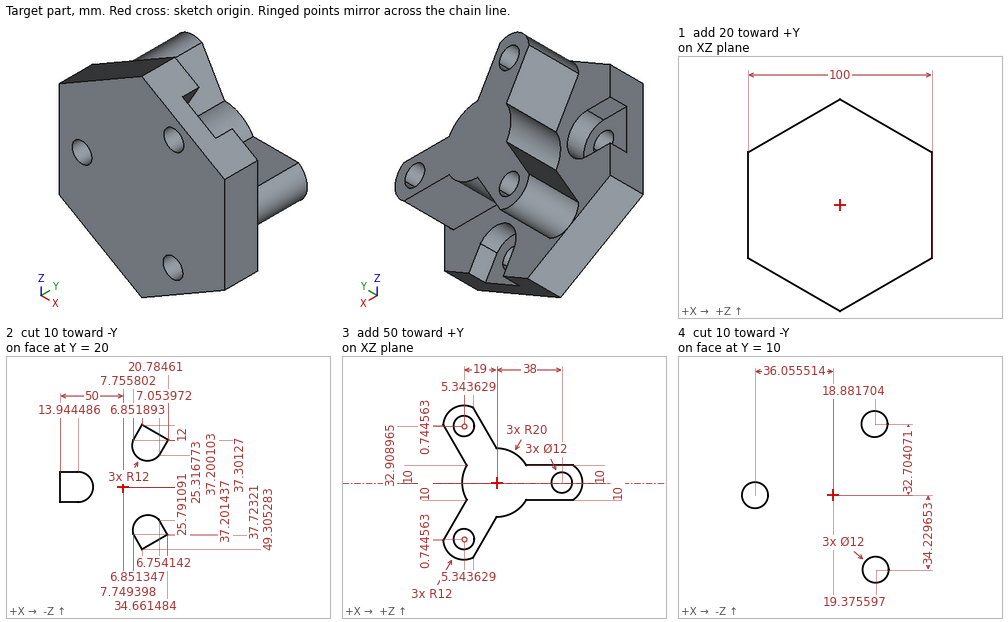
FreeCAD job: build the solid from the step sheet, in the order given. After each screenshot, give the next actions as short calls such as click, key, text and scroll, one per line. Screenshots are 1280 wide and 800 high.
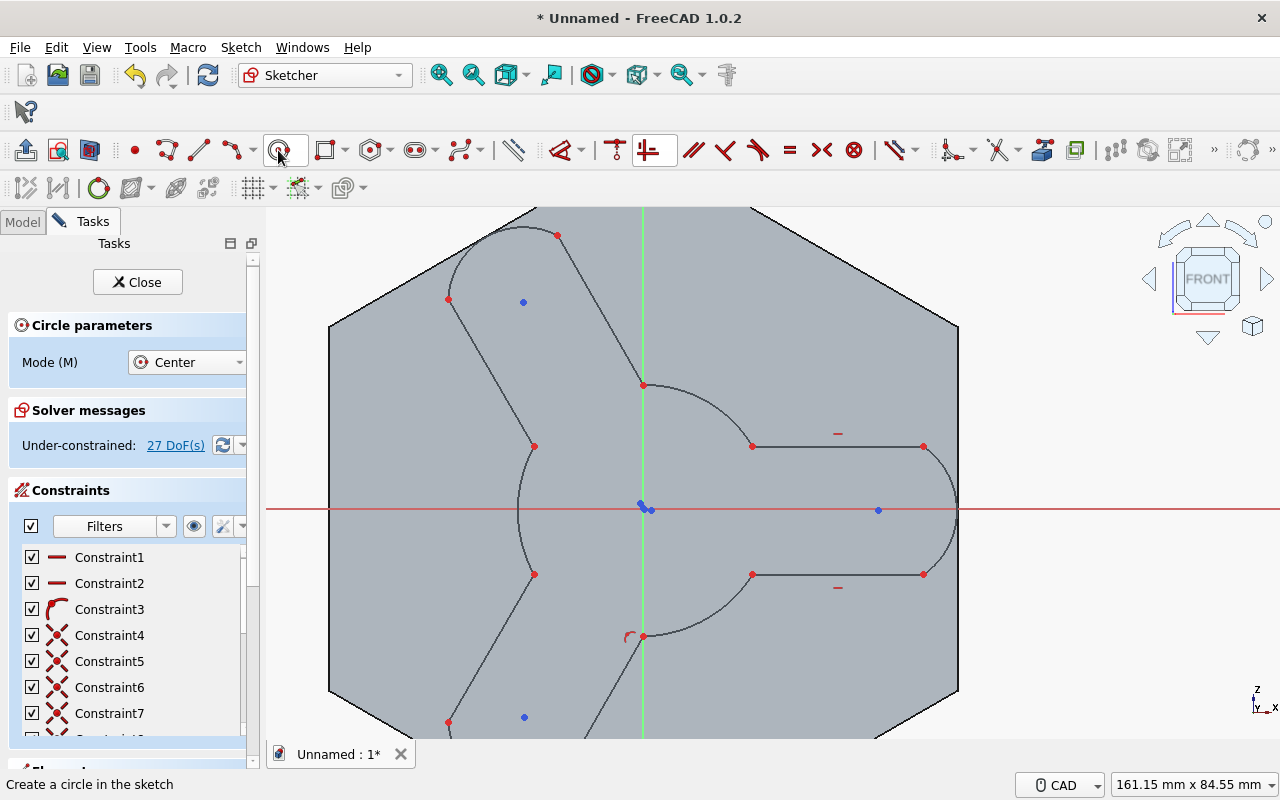
click(524, 302)
move(550, 275)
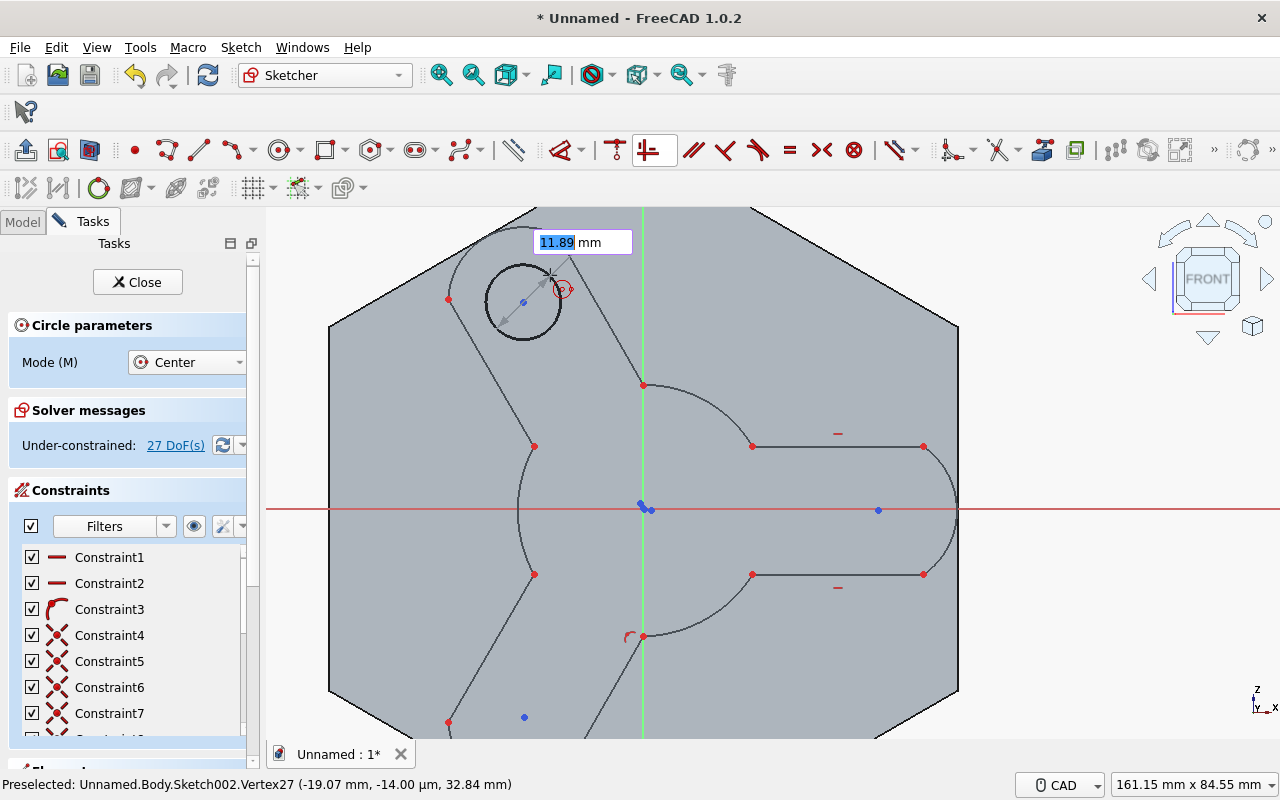
text(12)
key(Return)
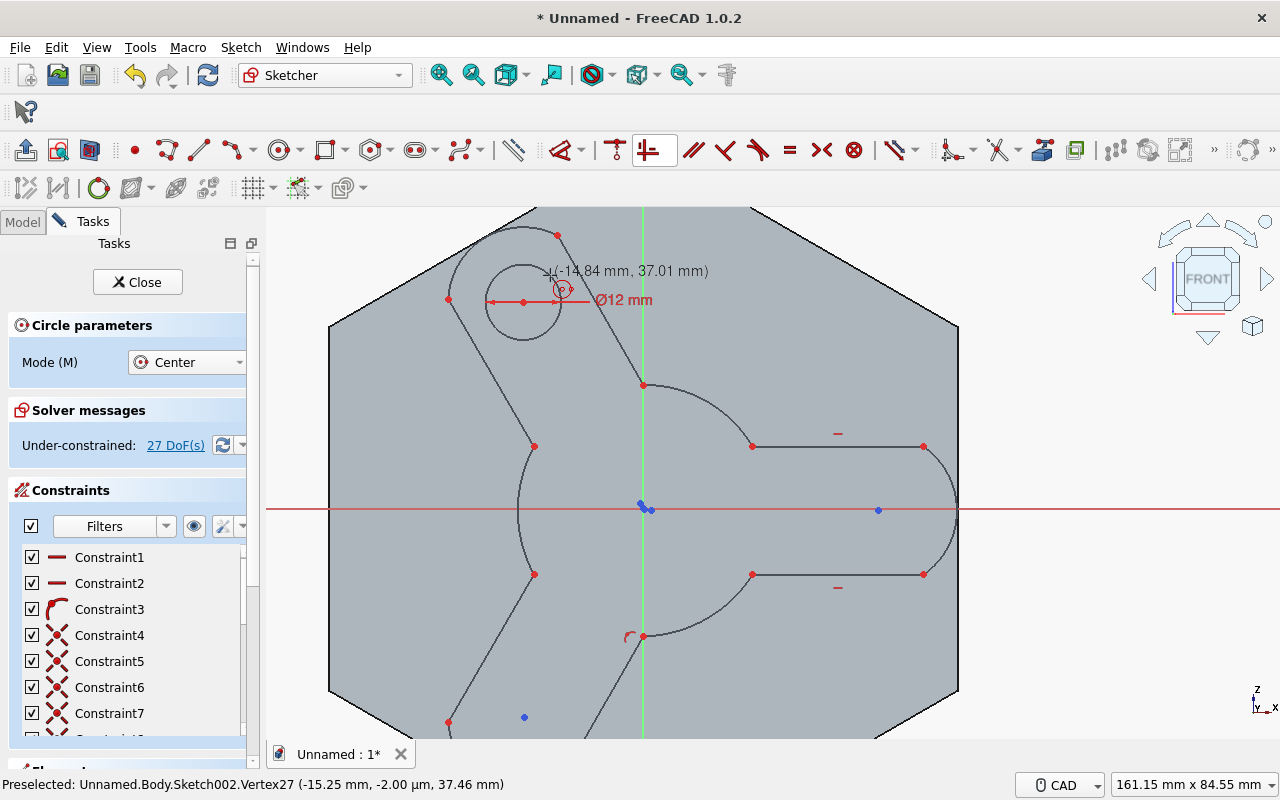
scroll(707, 400, down, 2)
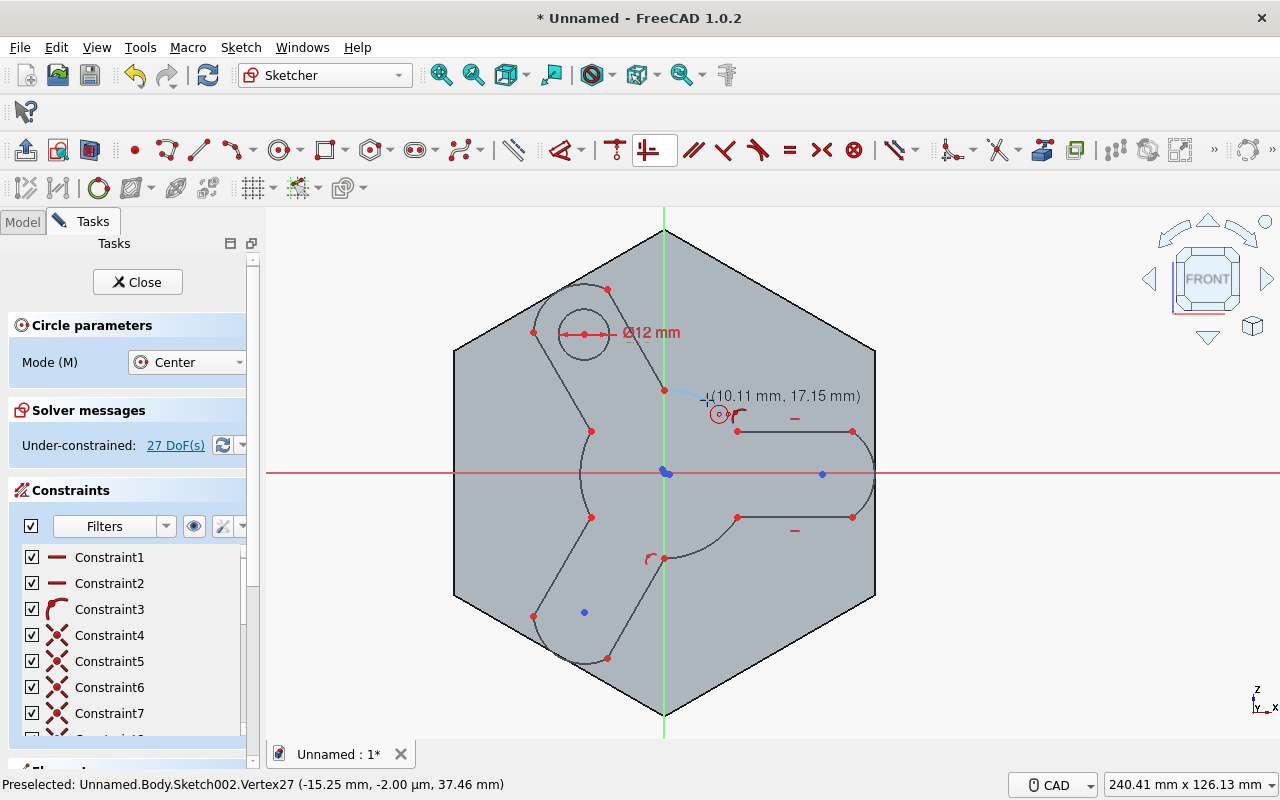
click(584, 612)
move(602, 594)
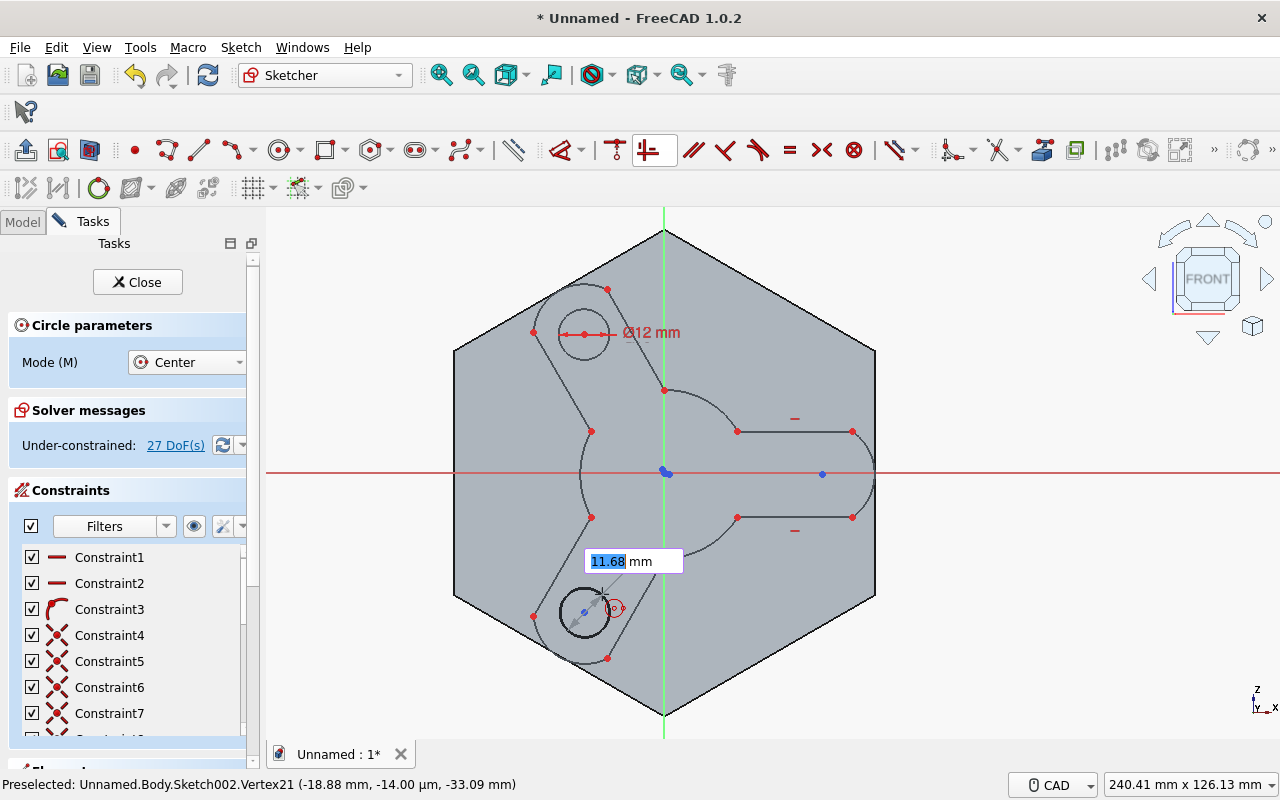
text(12)
key(Return)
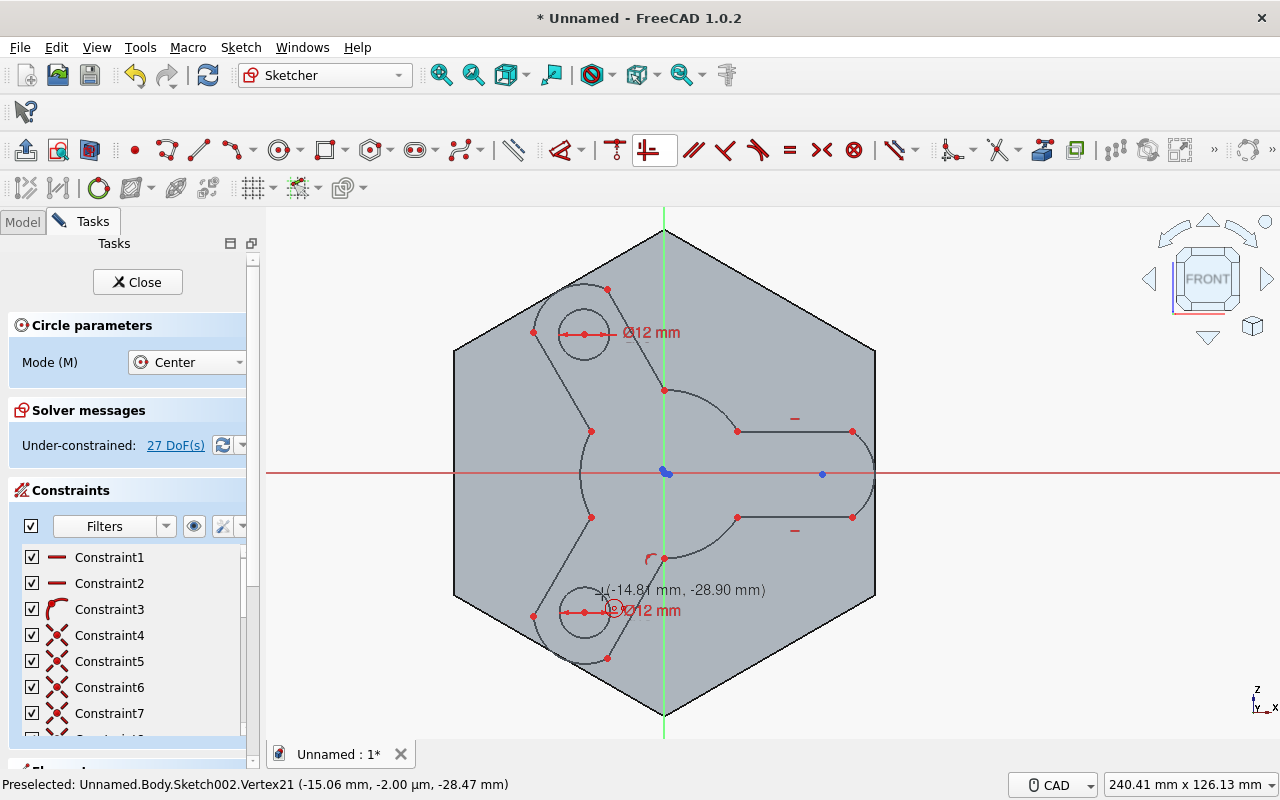
click(825, 473)
move(843, 455)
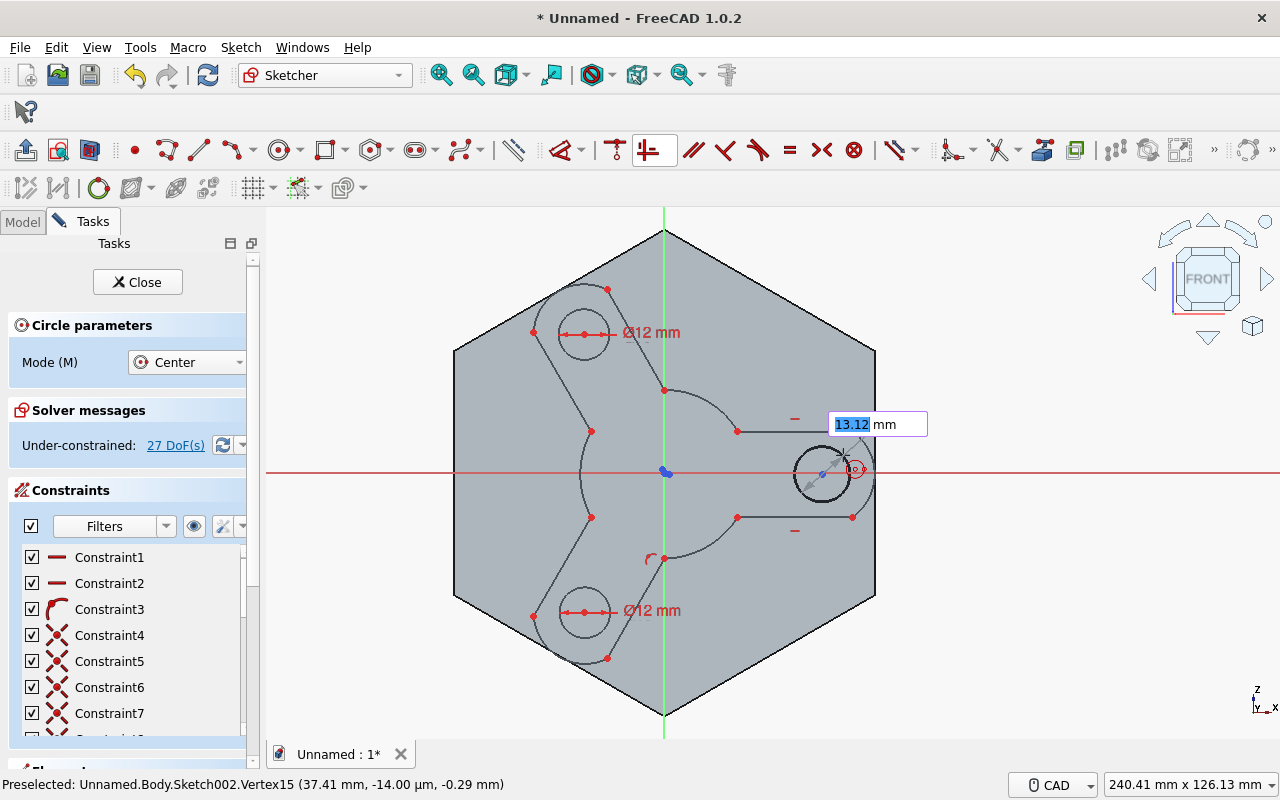
text(12)
key(Return)
key(Escape)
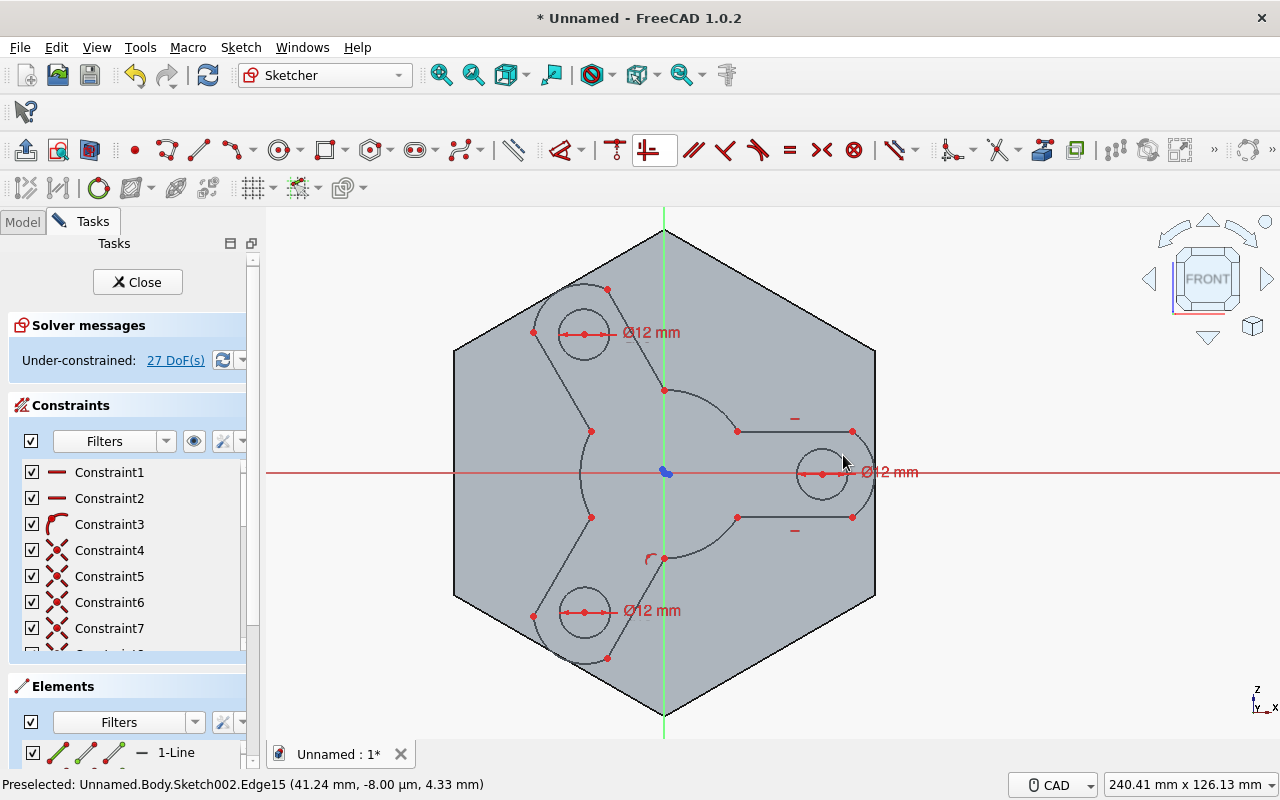
click(690, 554)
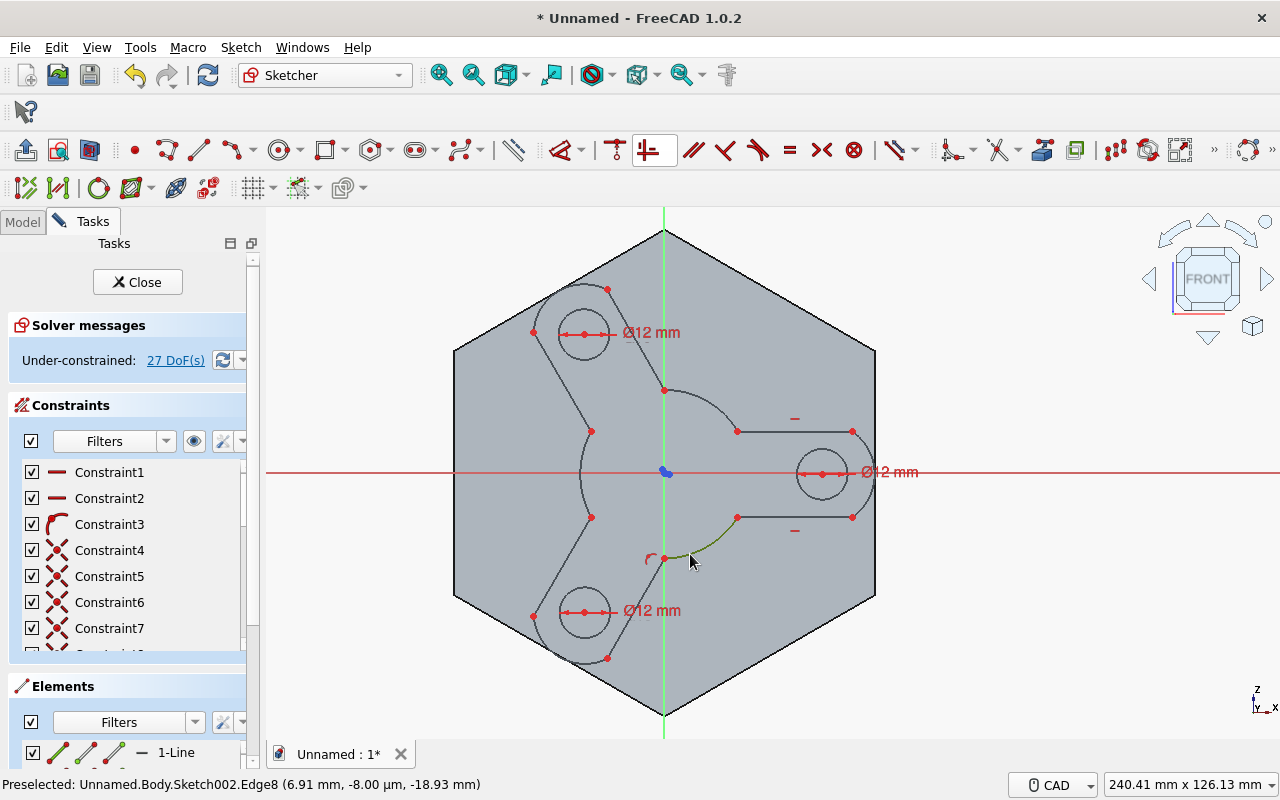
click(582, 457)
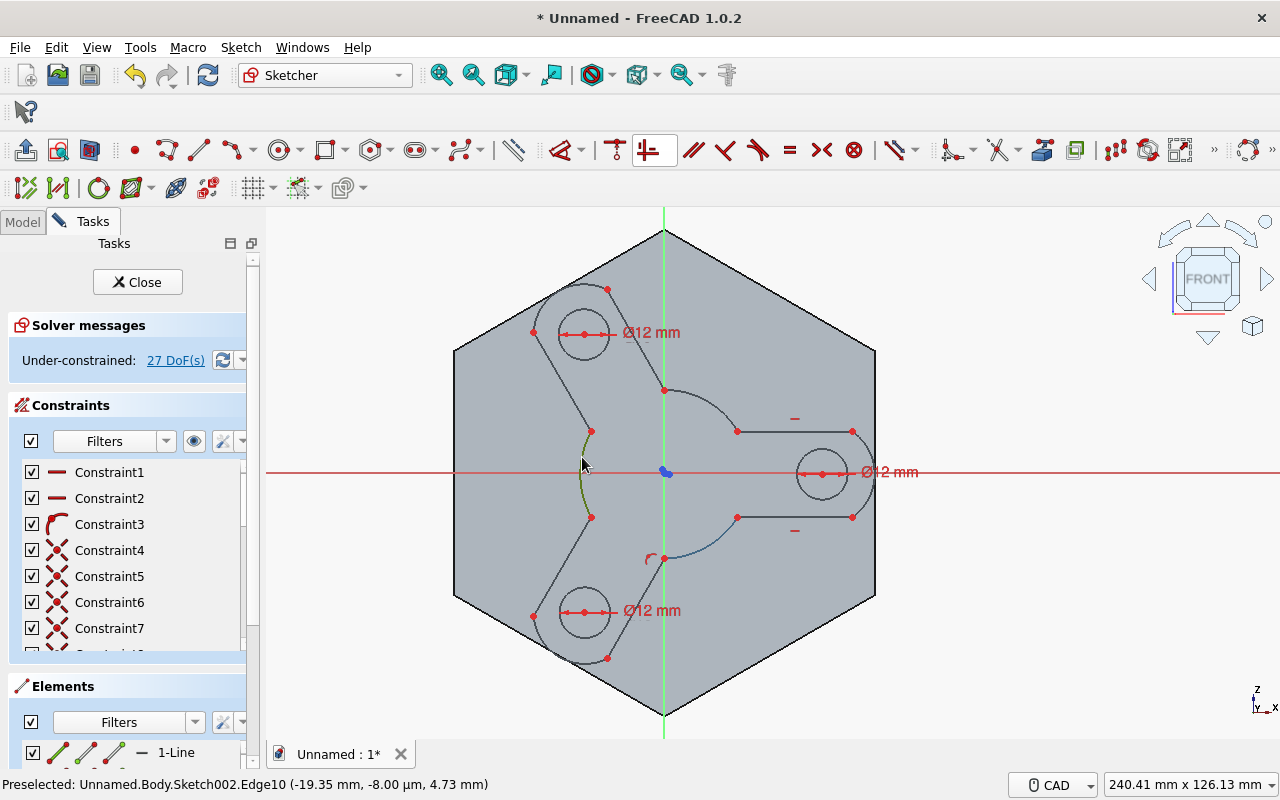
click(616, 150)